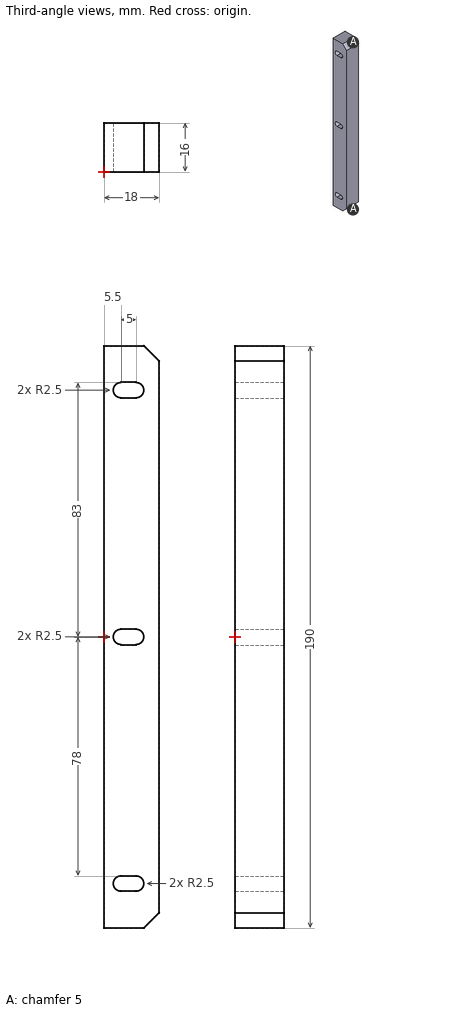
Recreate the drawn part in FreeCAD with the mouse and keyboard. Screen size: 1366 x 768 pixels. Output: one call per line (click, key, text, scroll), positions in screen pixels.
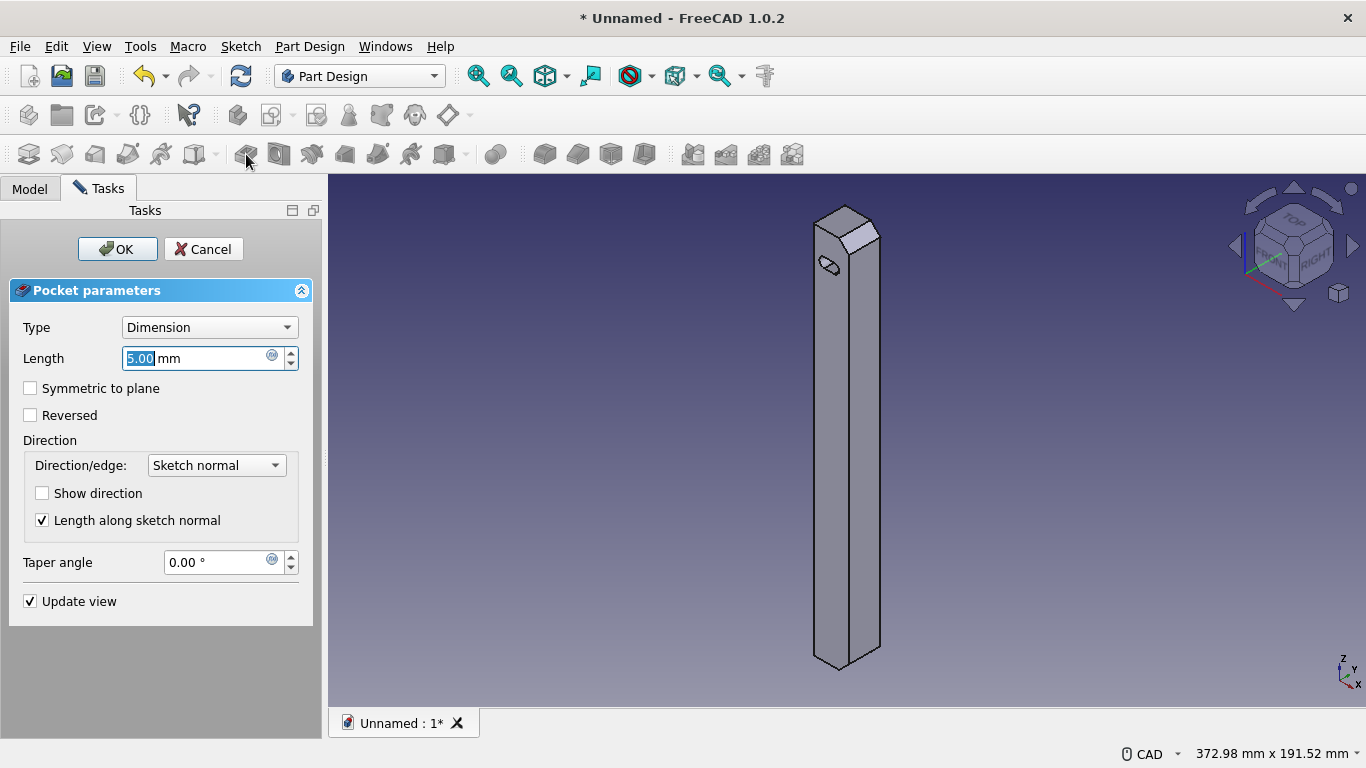
click(210, 328)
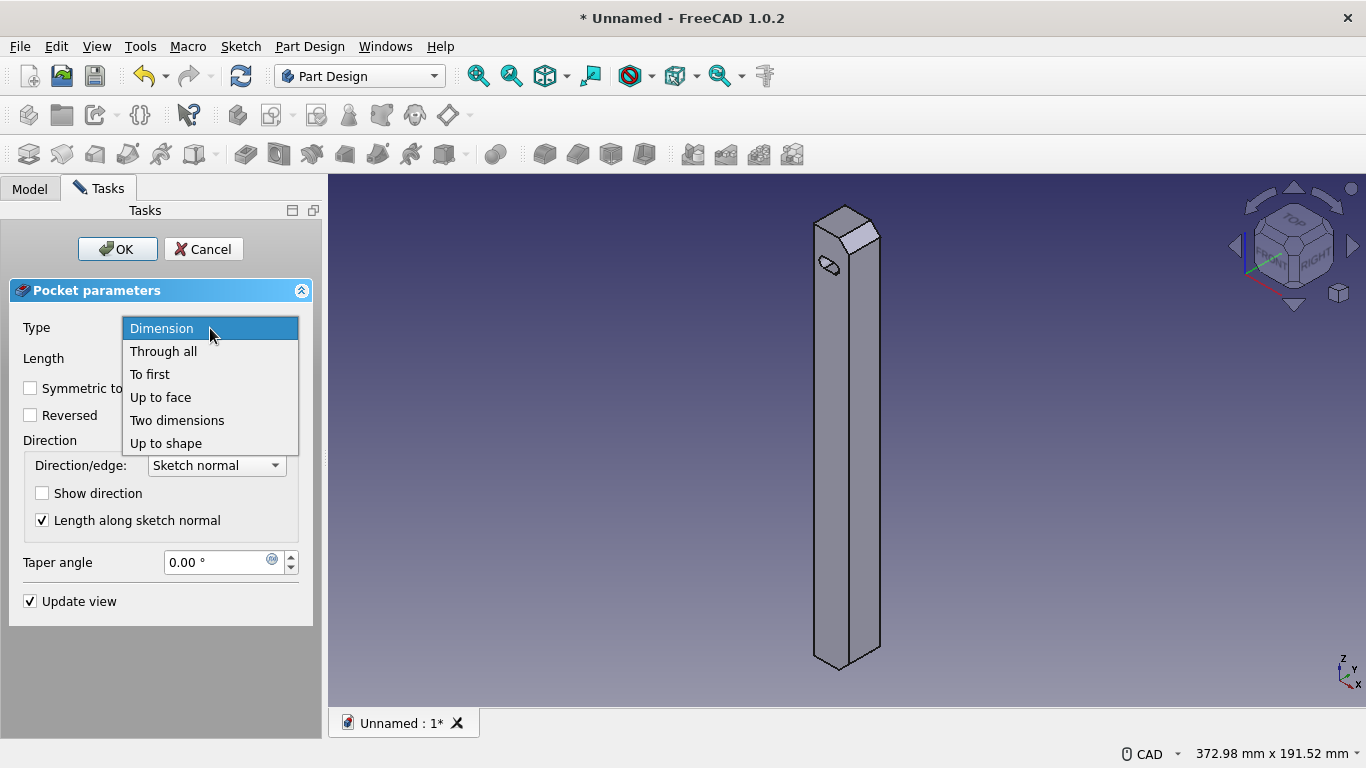
click(208, 374)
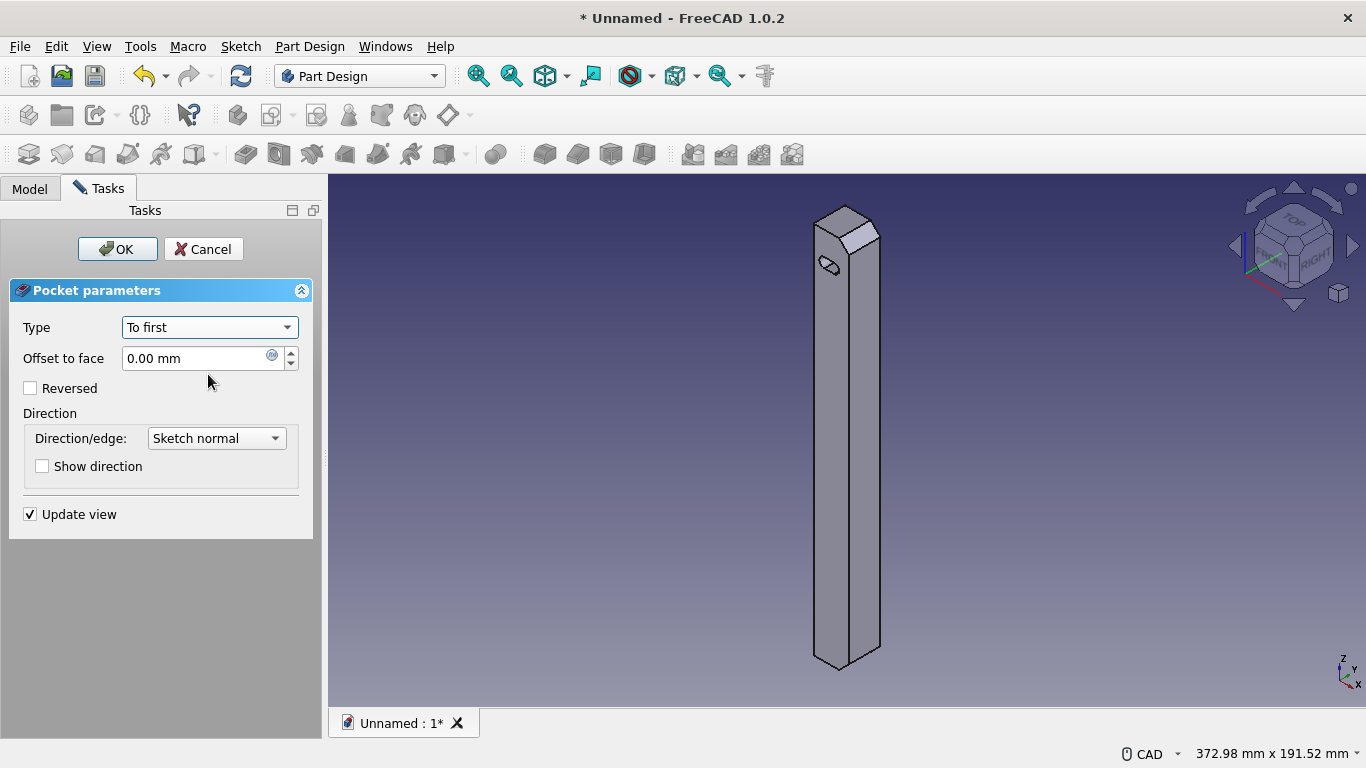
click(118, 249)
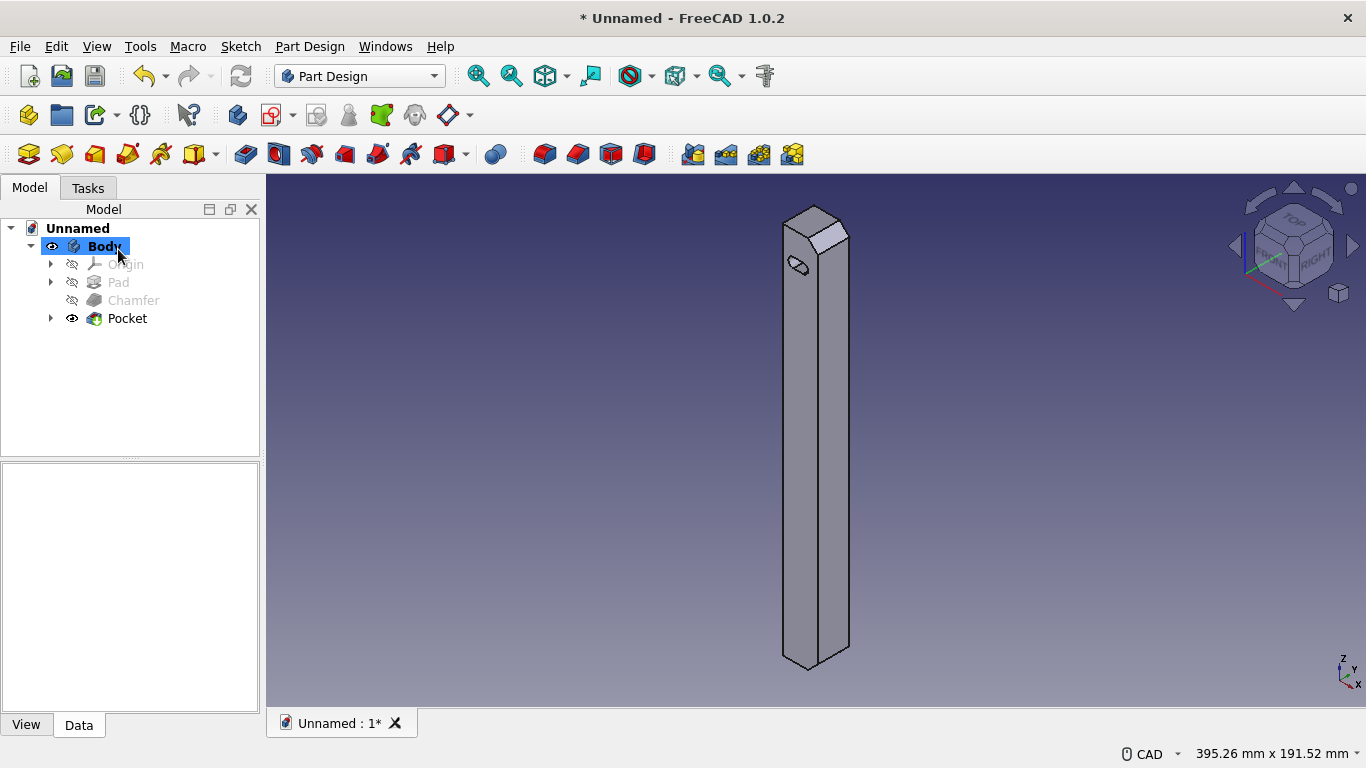
click(270, 116)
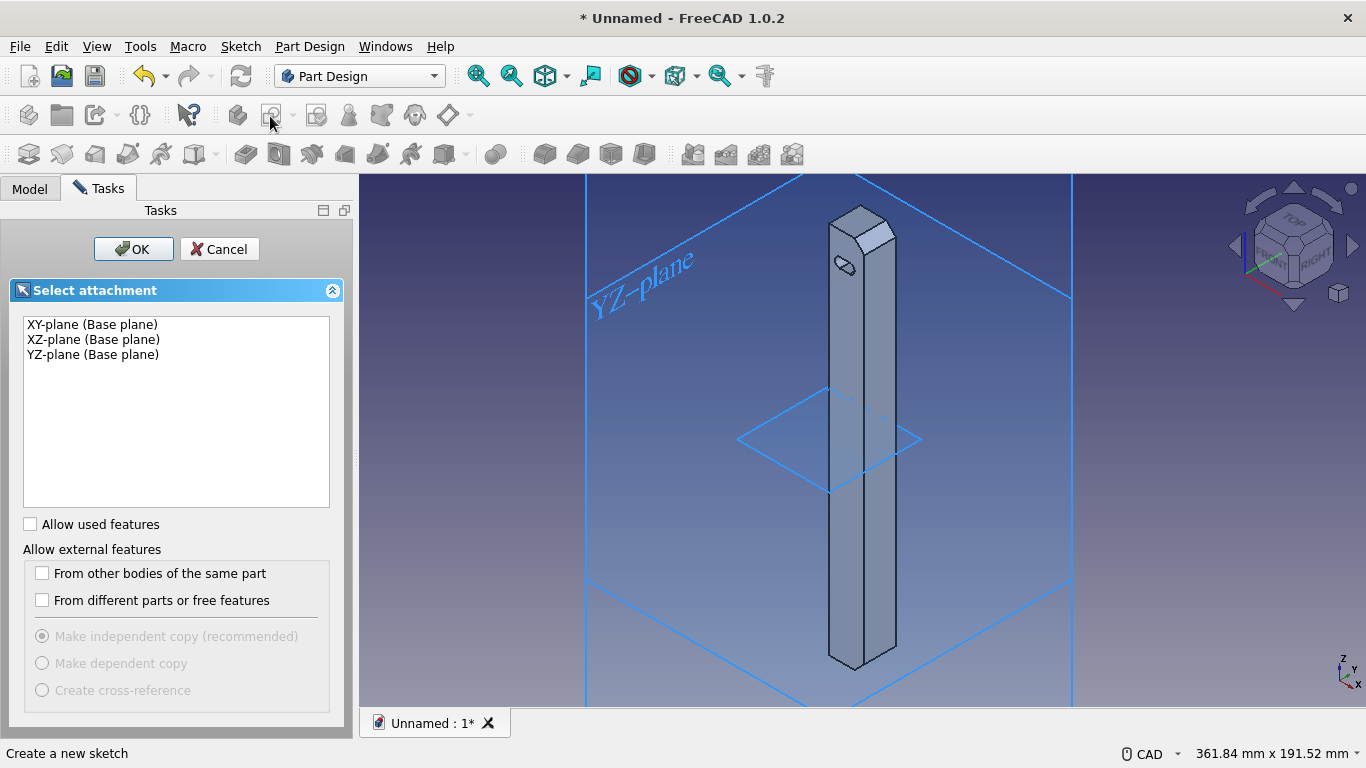
click(84, 340)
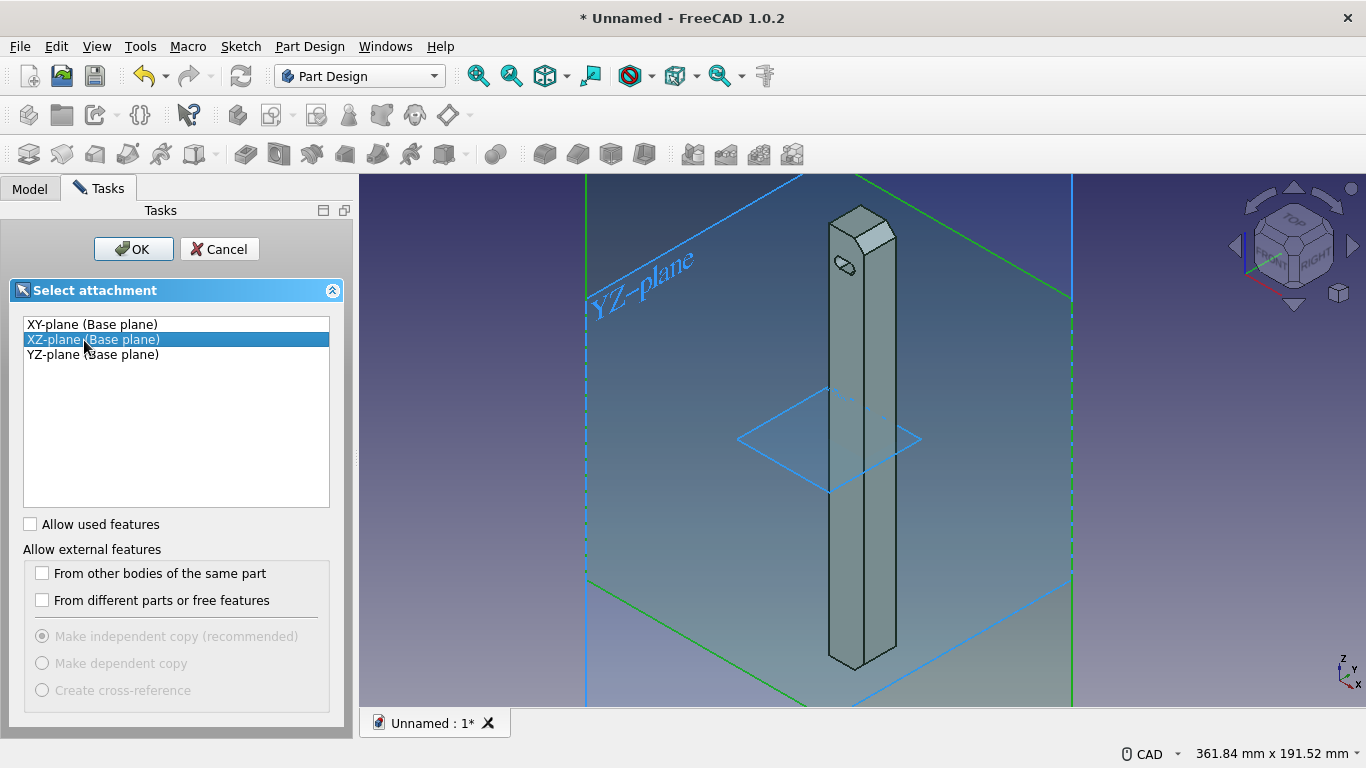
click(134, 249)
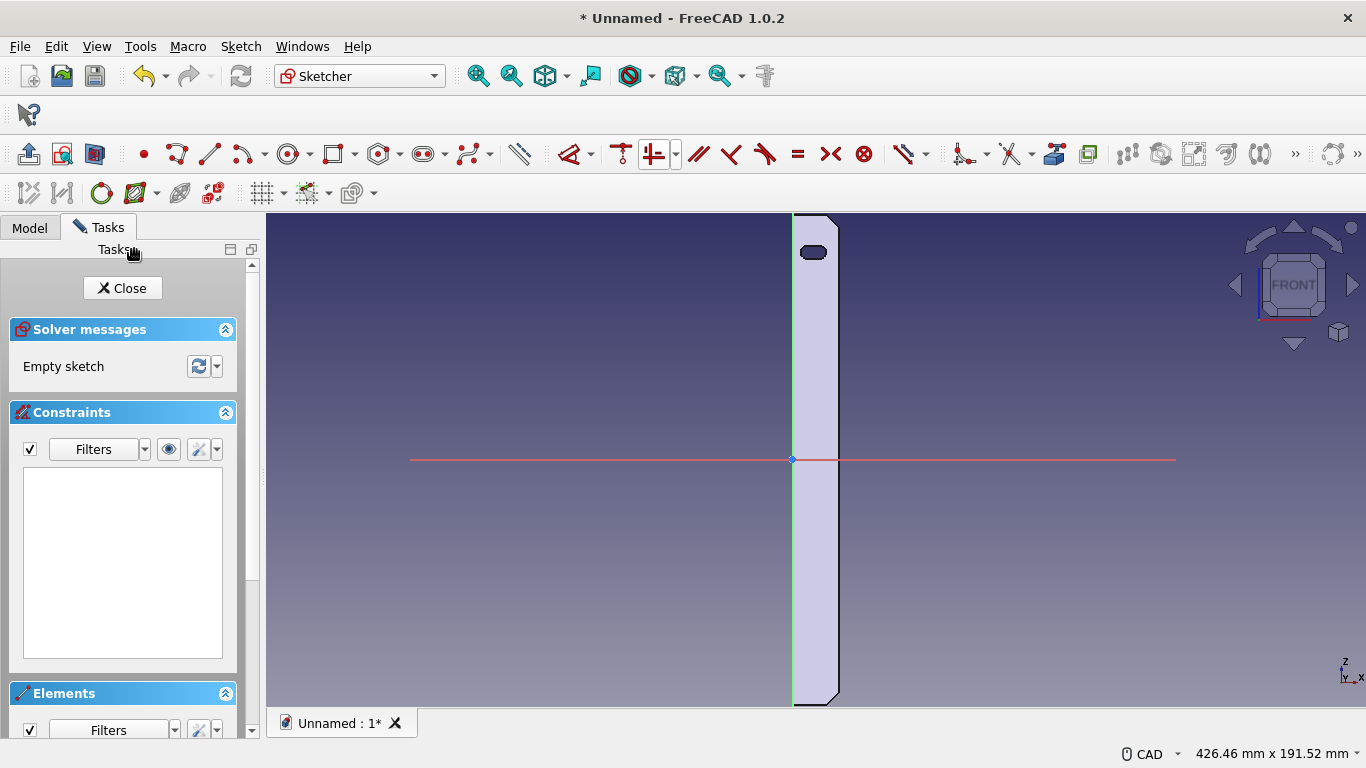
scroll(813, 460, up, 15)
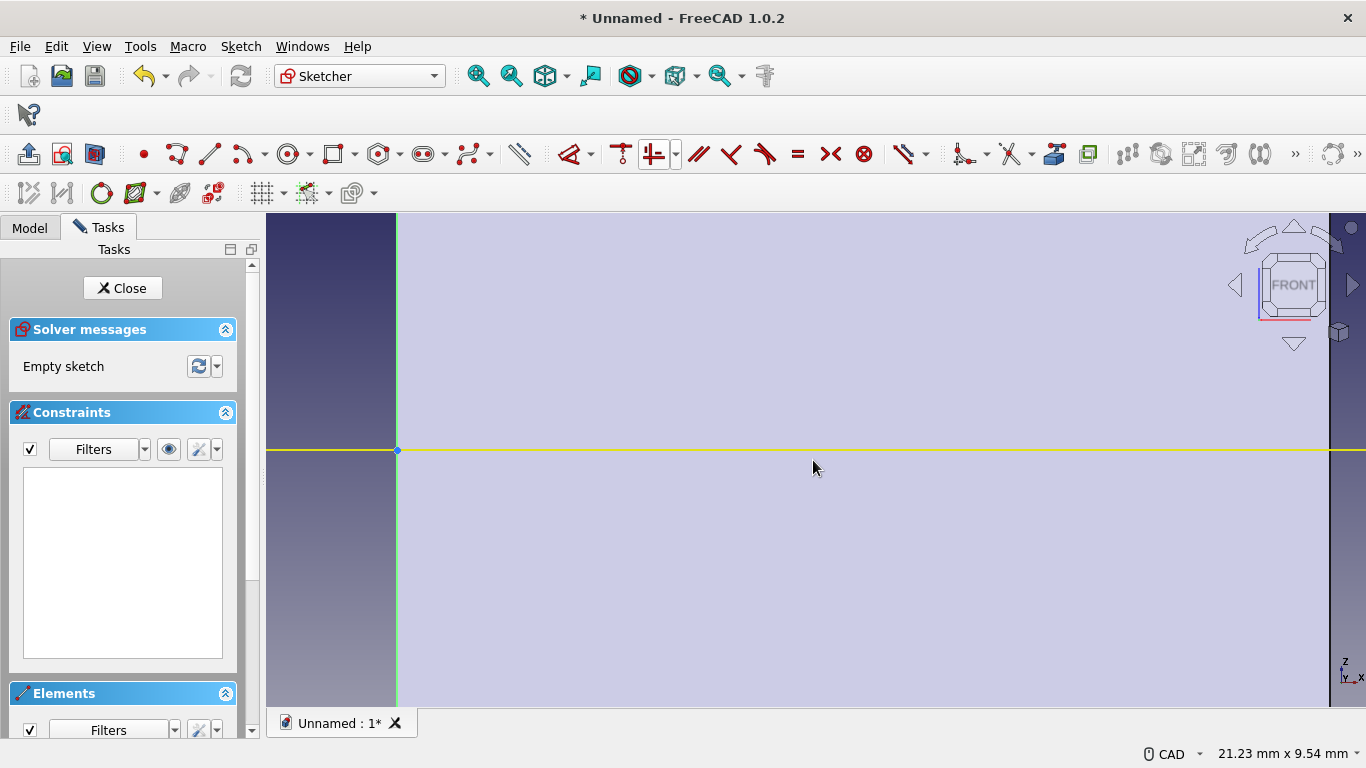
click(422, 154)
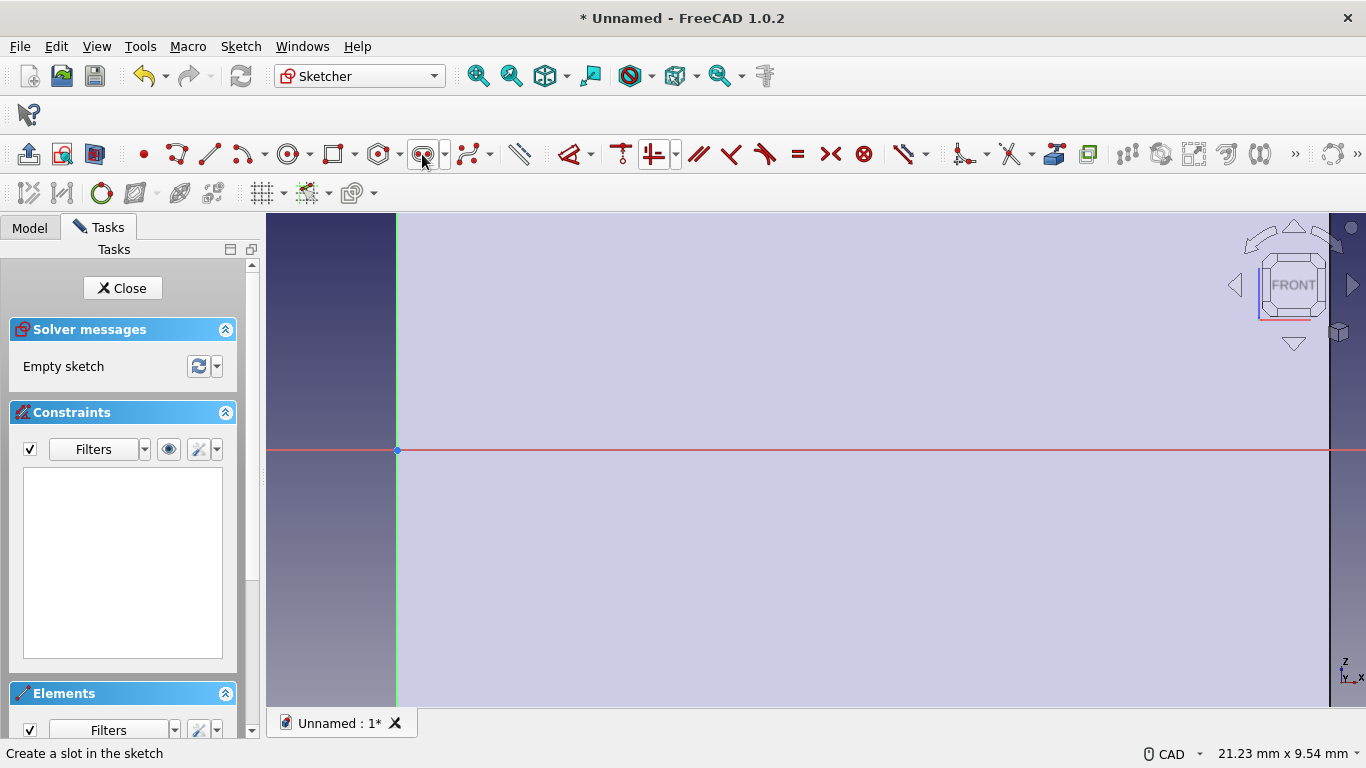
click(682, 450)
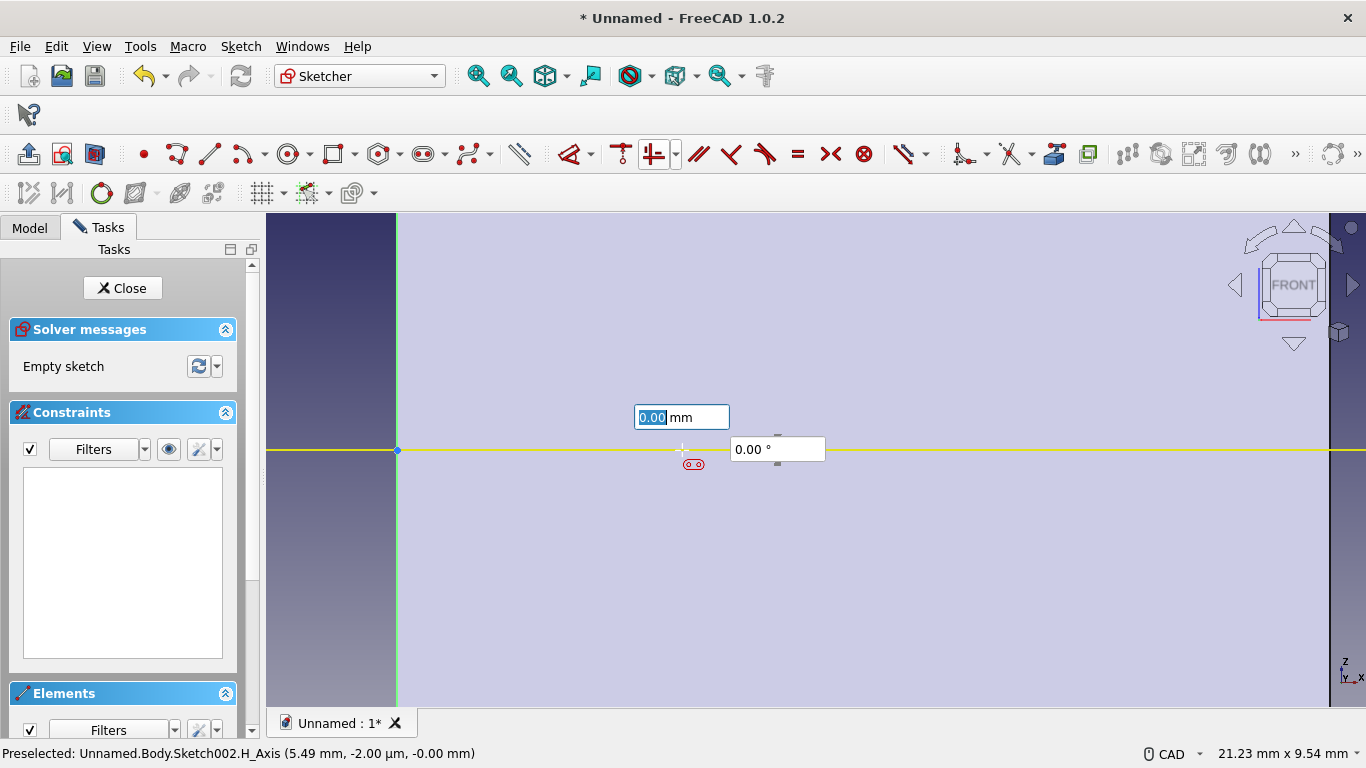
click(941, 441)